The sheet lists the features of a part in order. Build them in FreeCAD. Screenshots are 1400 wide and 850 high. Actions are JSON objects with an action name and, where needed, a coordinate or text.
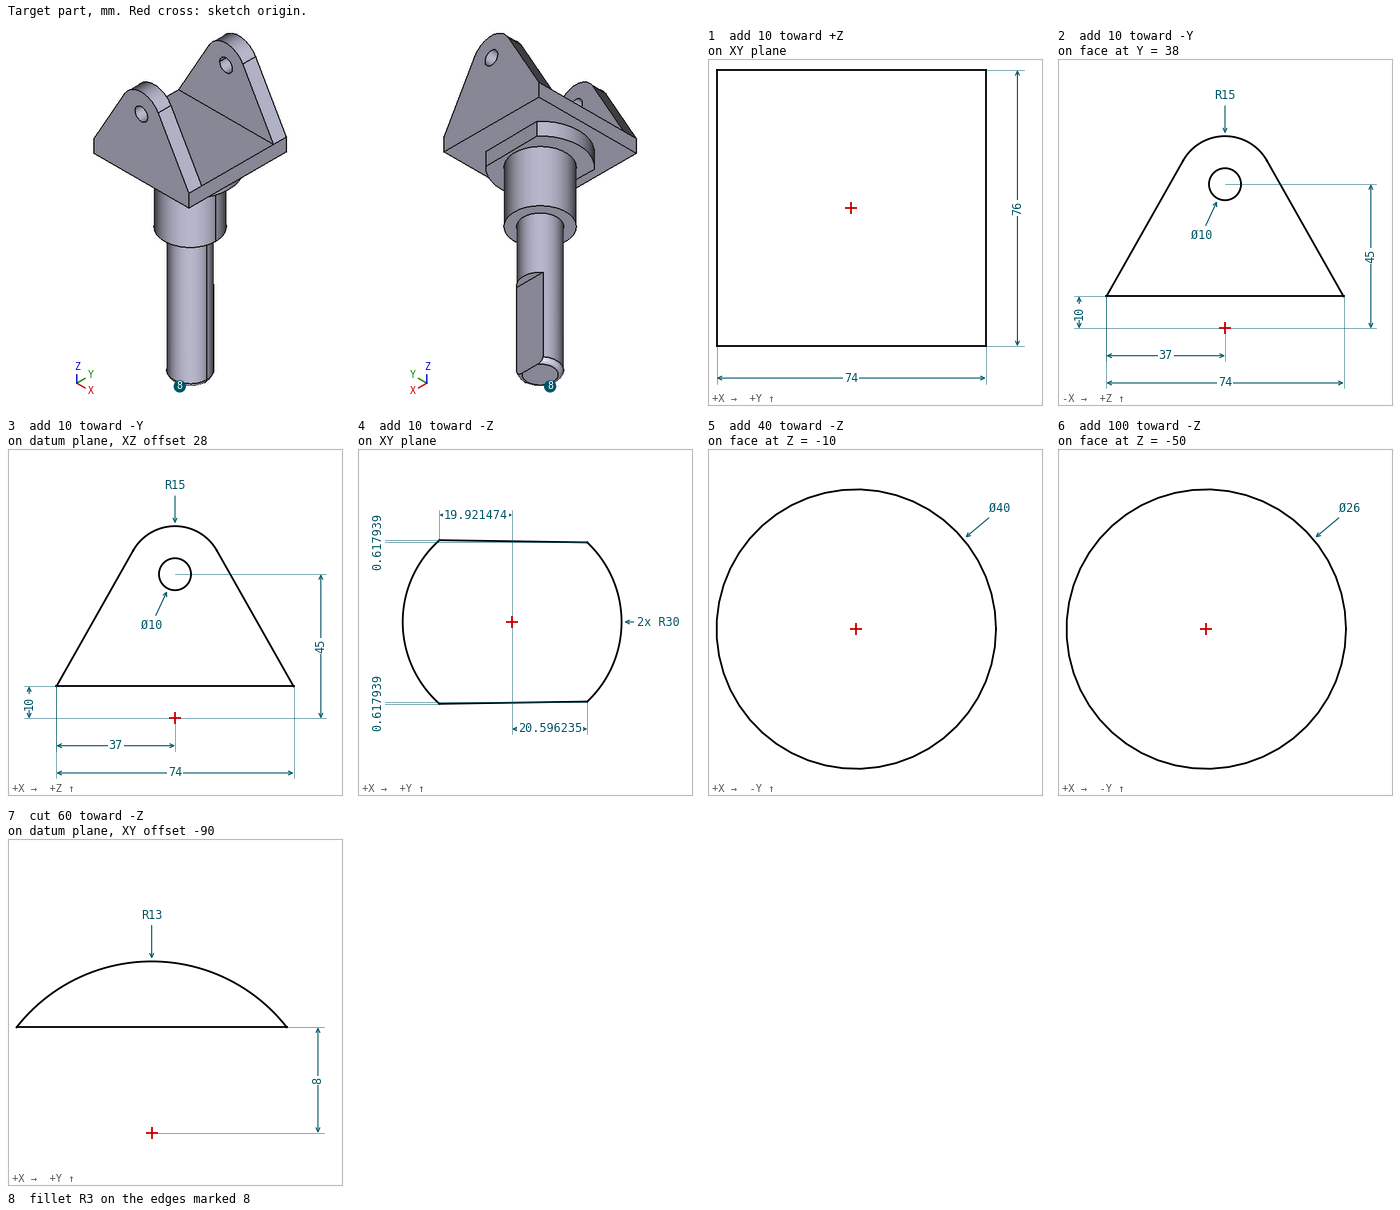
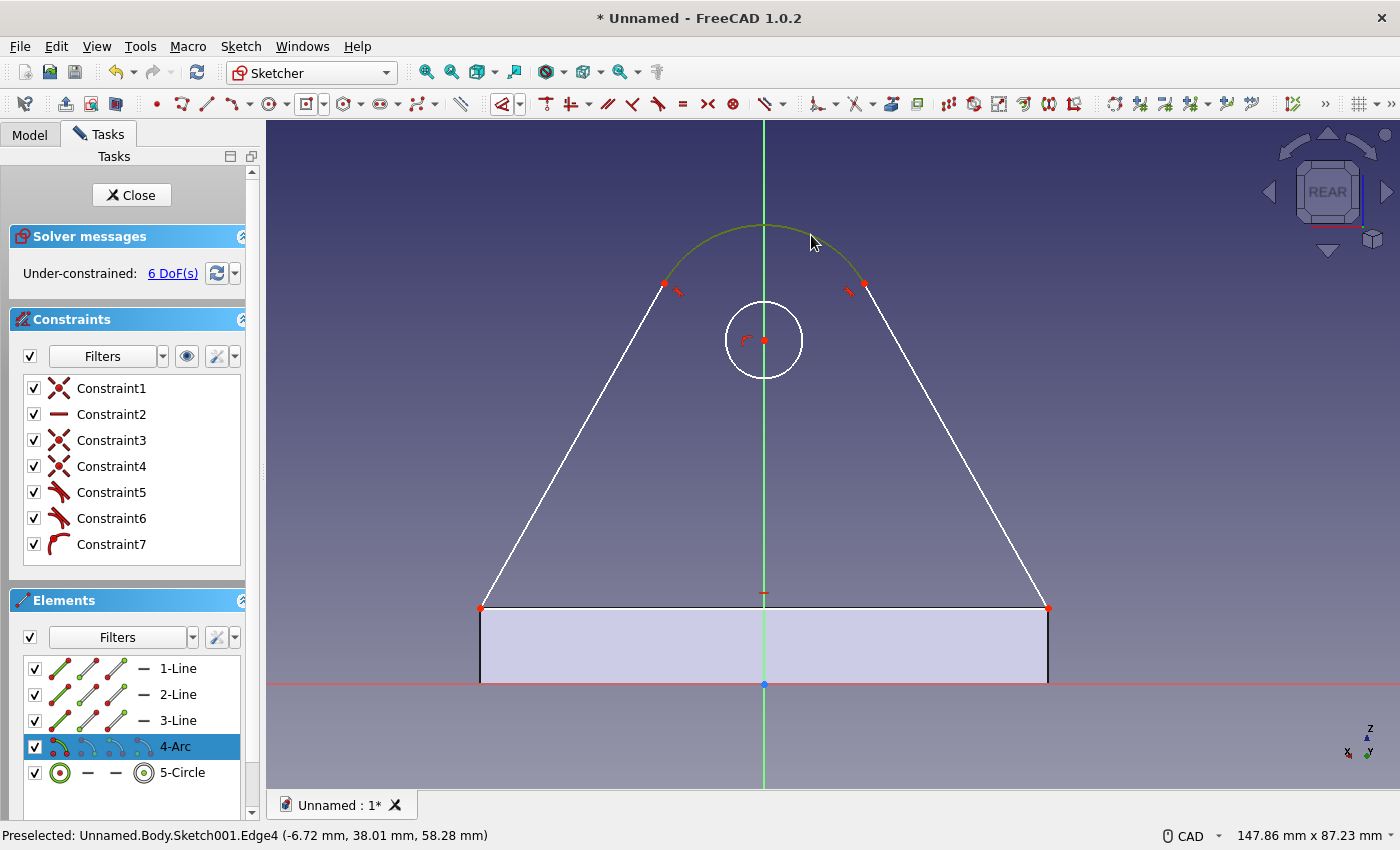
{"action": "left_click", "coordinate": [520, 104]}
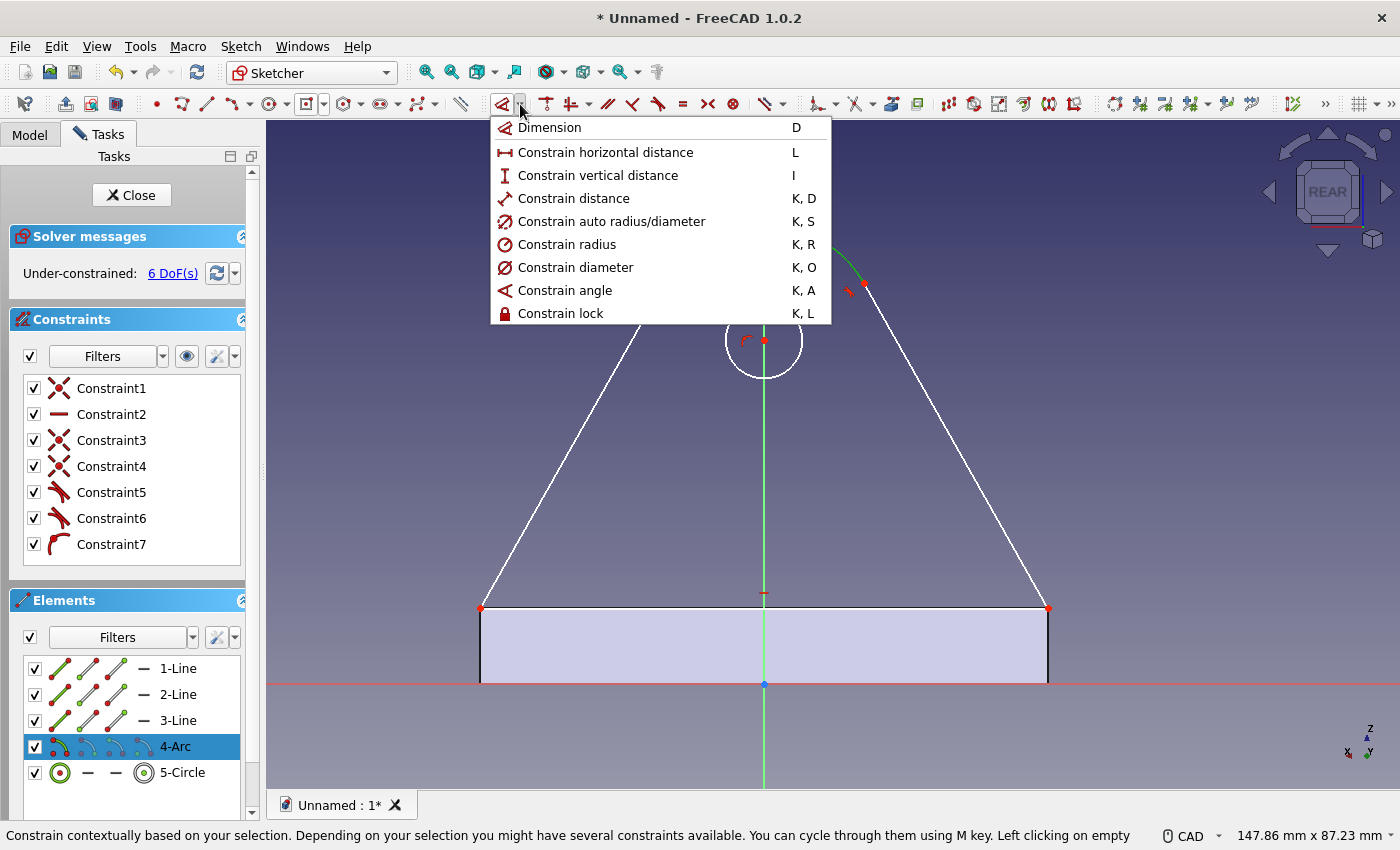
{"action": "left_click", "coordinate": [661, 244]}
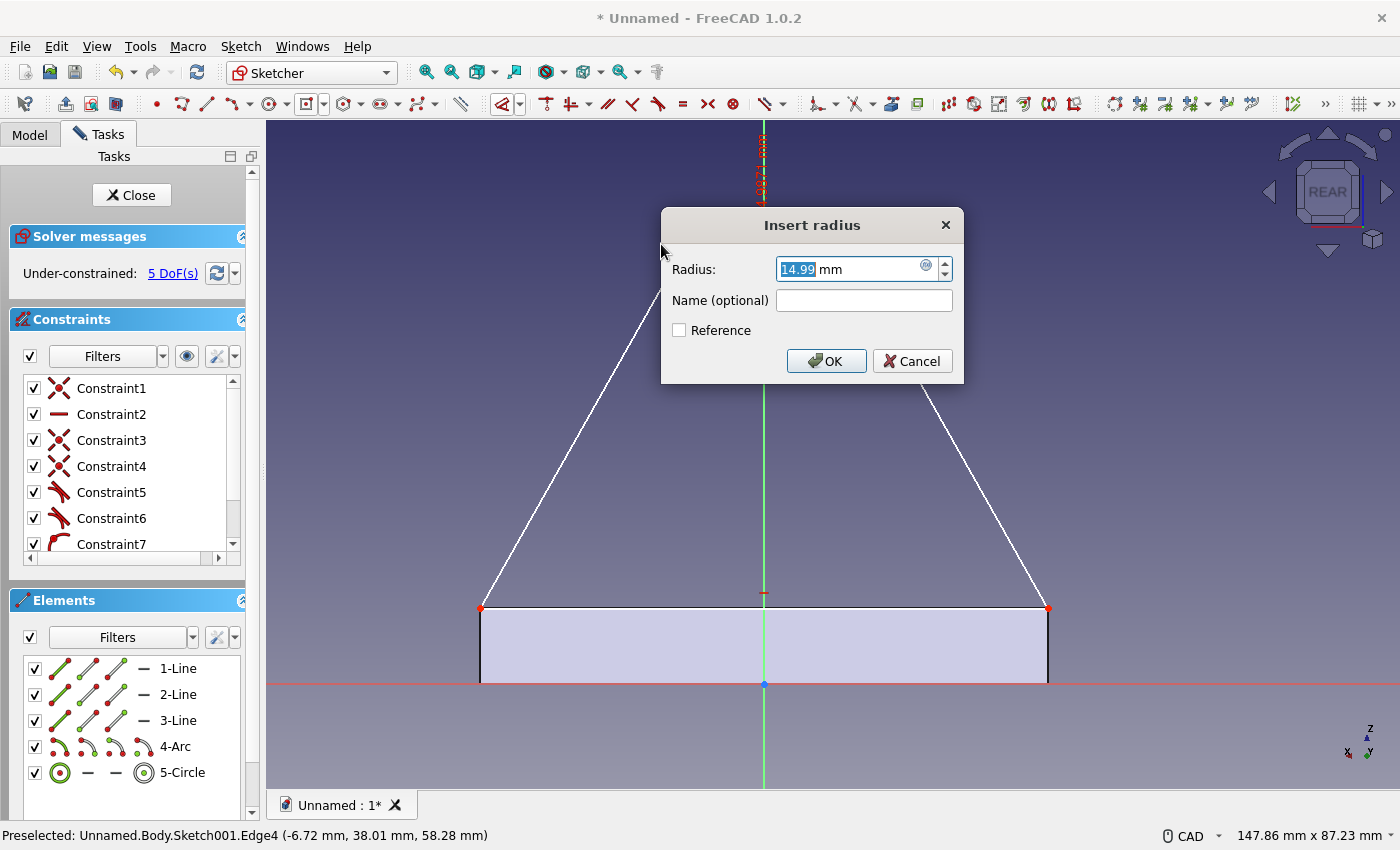
{"action": "type", "text": "15"}
{"action": "key", "text": "Return"}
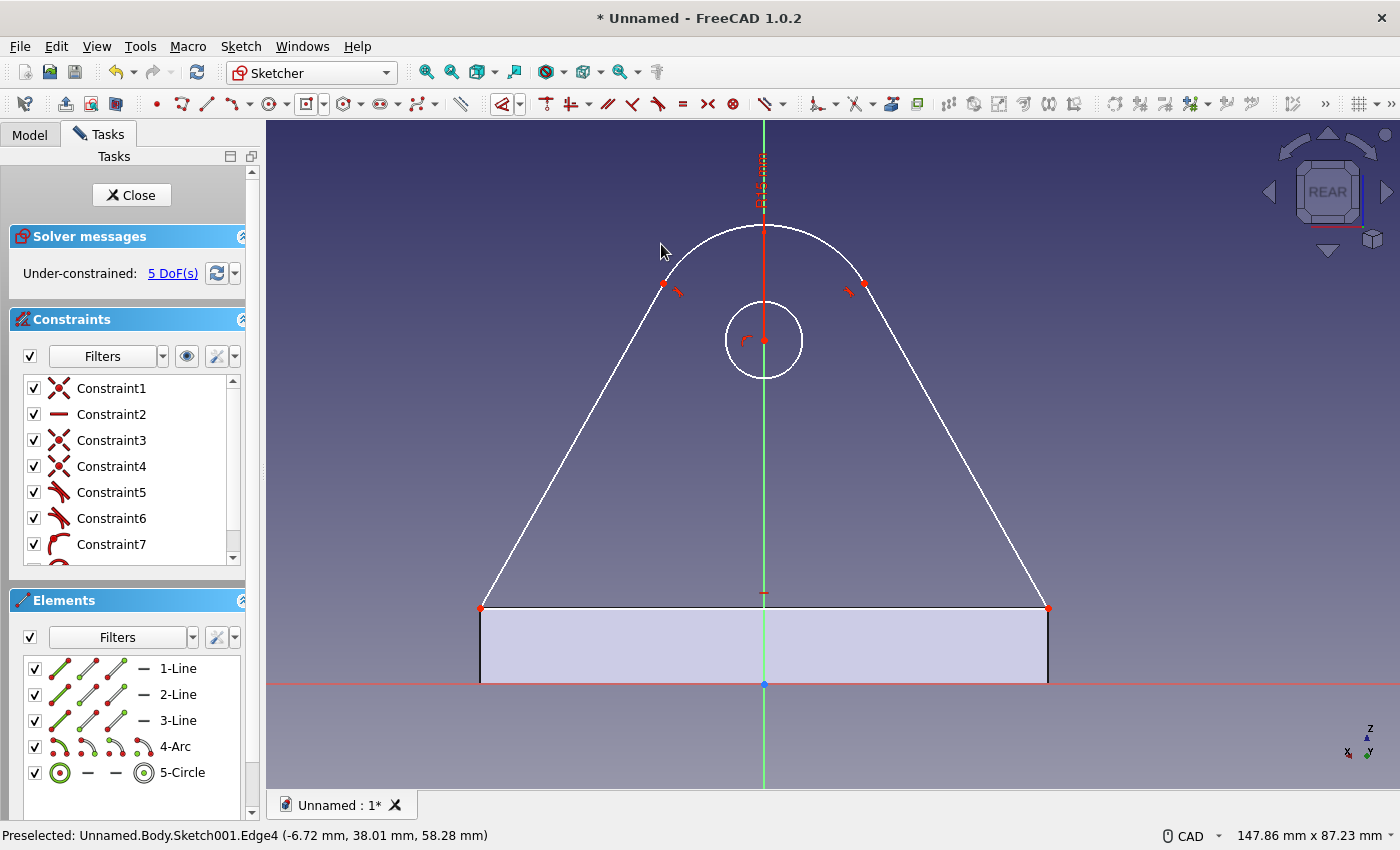
{"action": "left_click", "coordinate": [791, 313]}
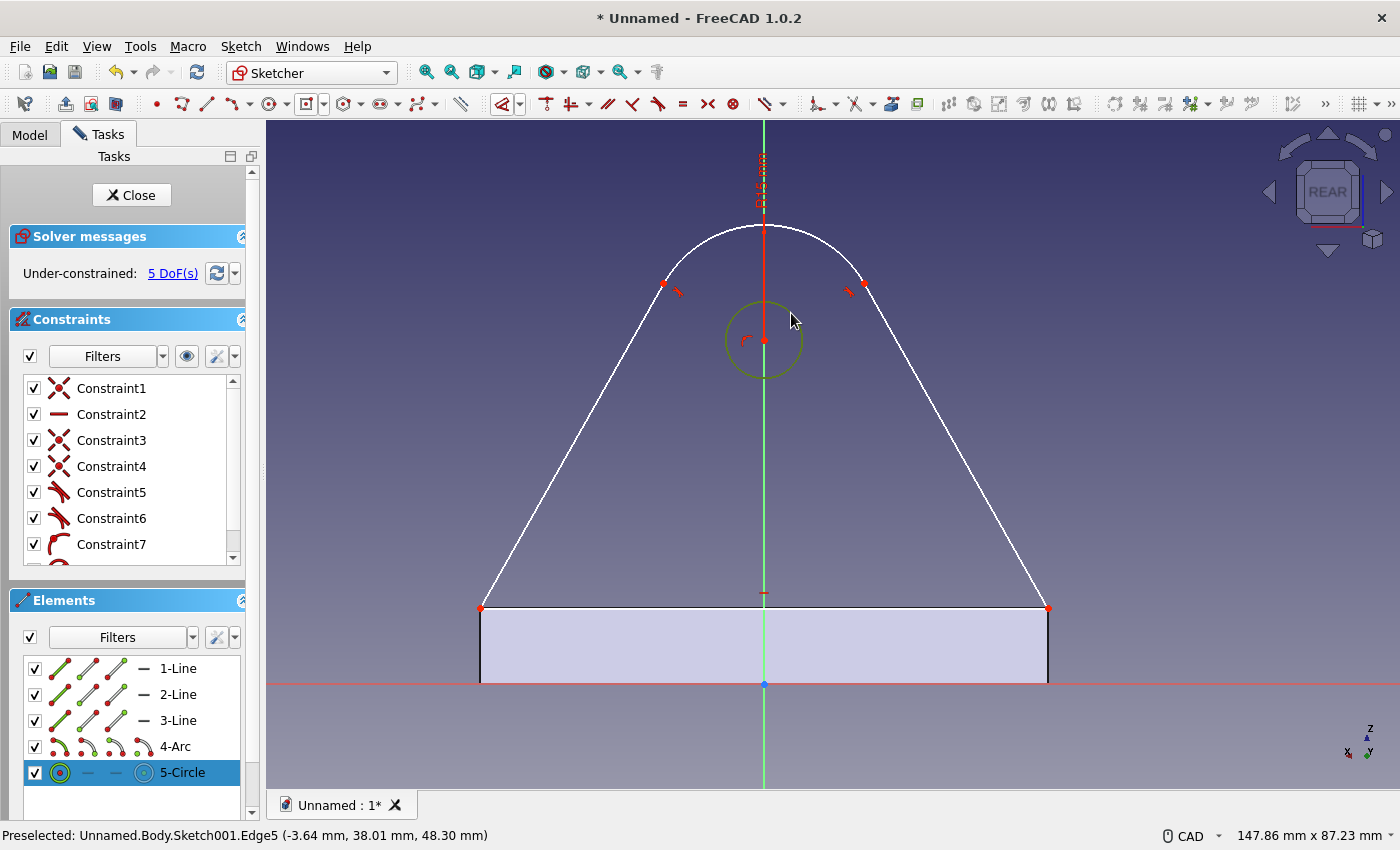
{"action": "left_click", "coordinate": [520, 104]}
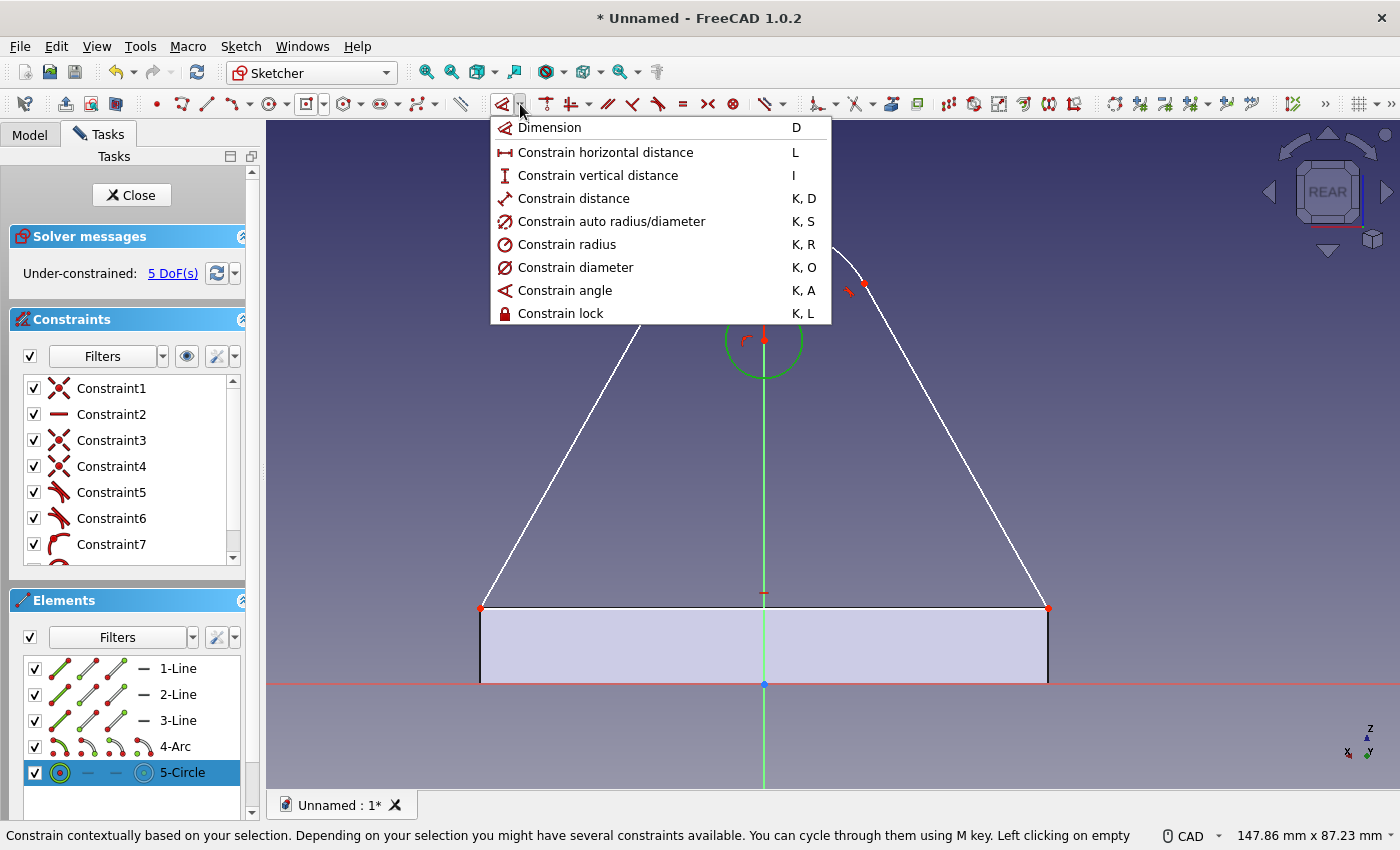
{"action": "left_click", "coordinate": [661, 268]}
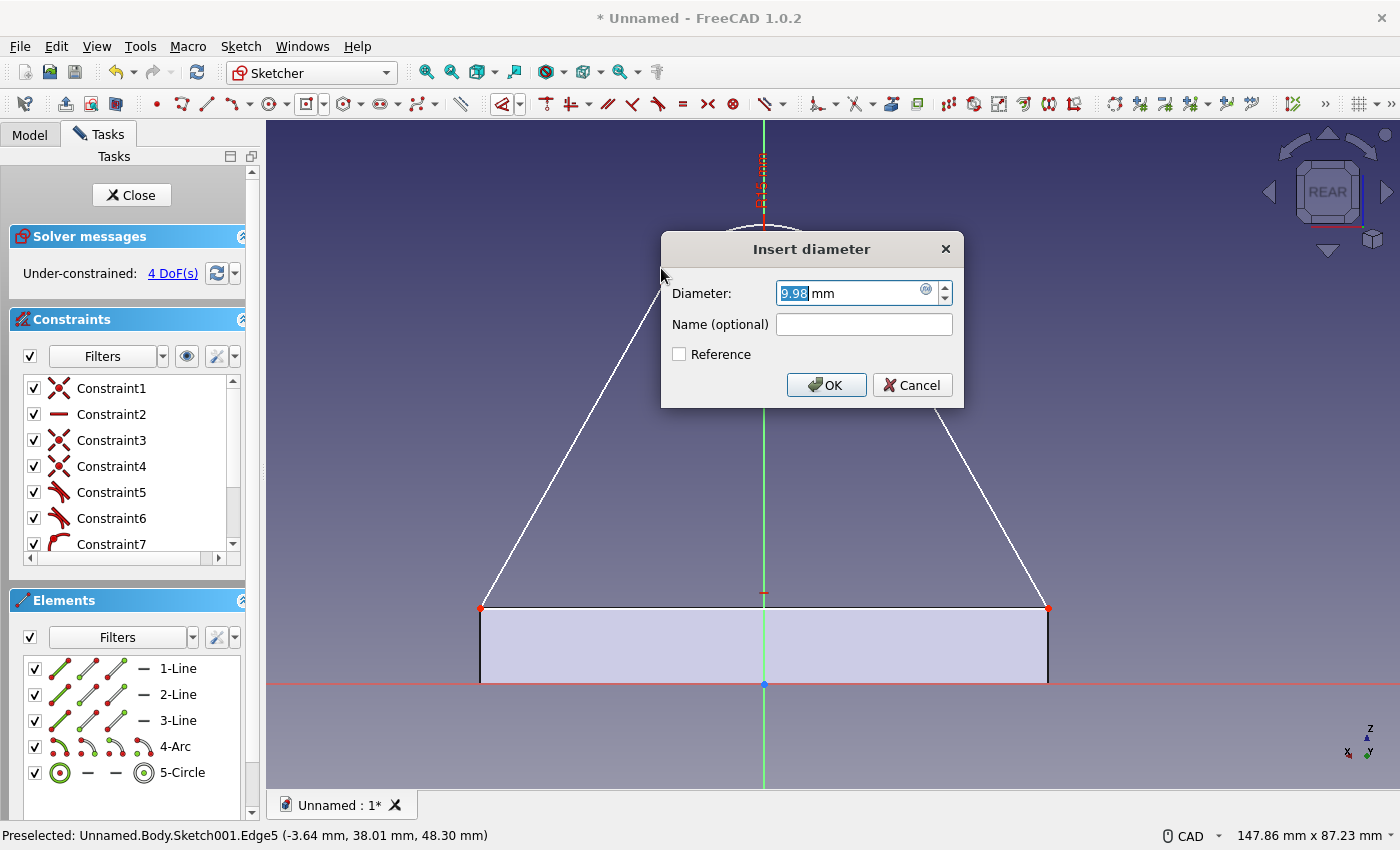
{"action": "type", "text": "10"}
{"action": "key", "text": "Return"}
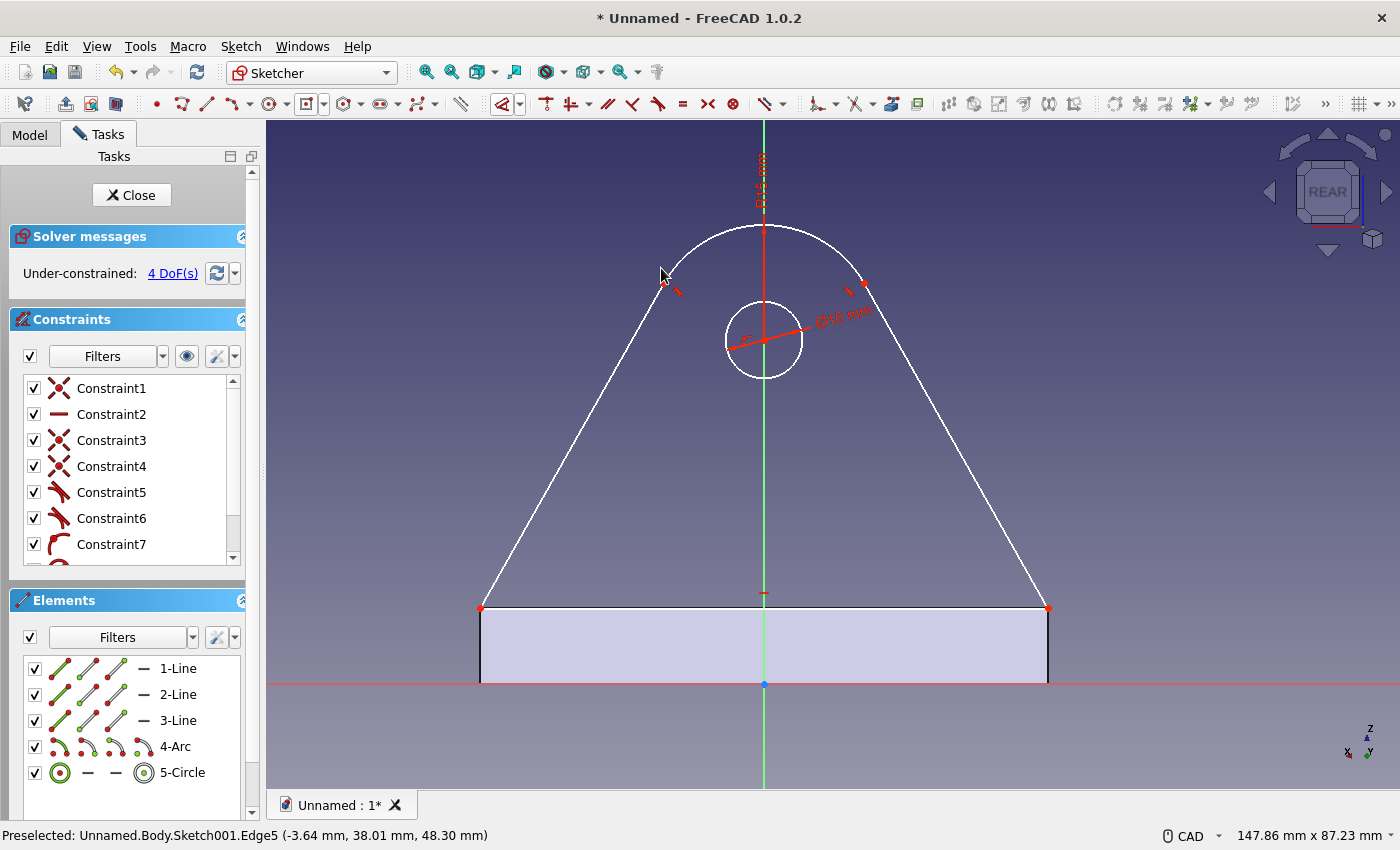
{"action": "left_click", "coordinate": [650, 609]}